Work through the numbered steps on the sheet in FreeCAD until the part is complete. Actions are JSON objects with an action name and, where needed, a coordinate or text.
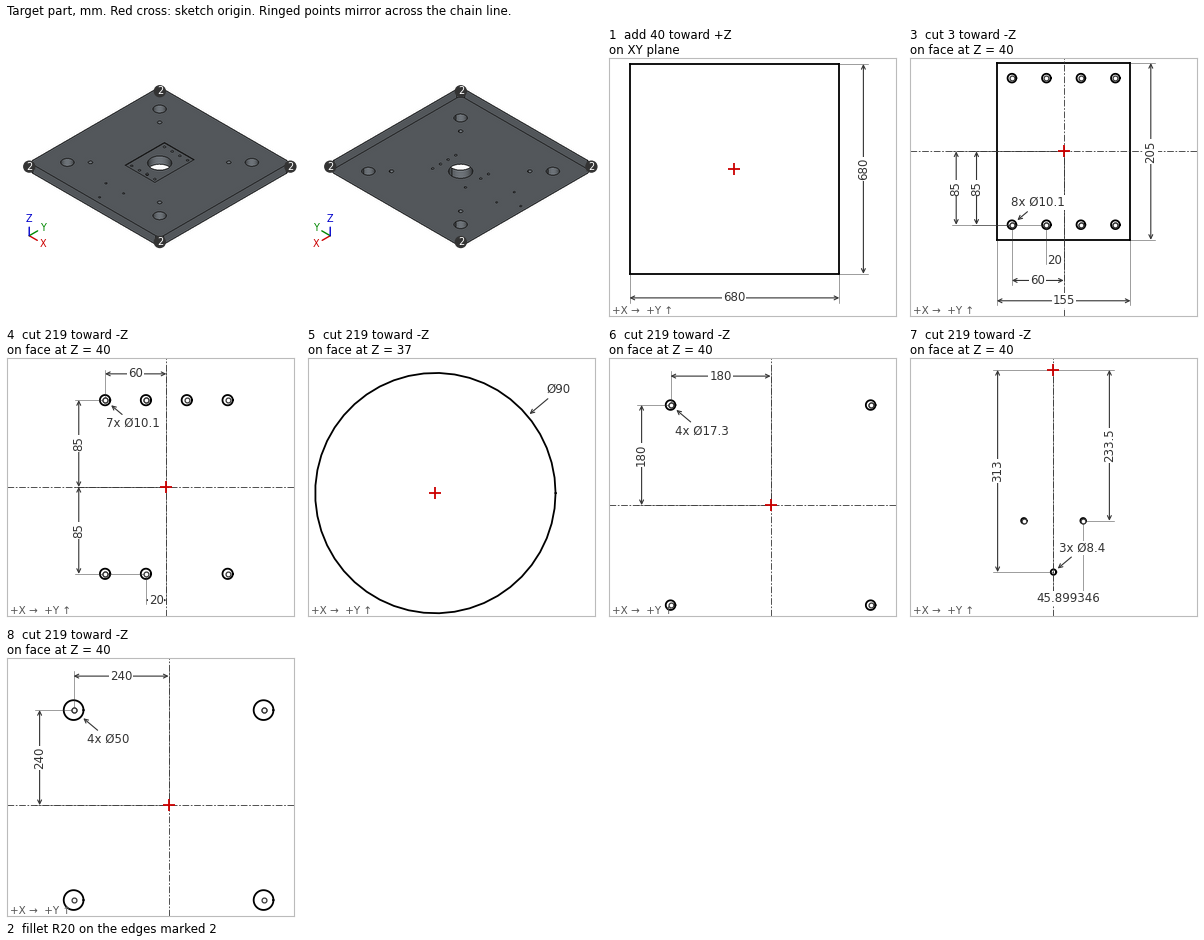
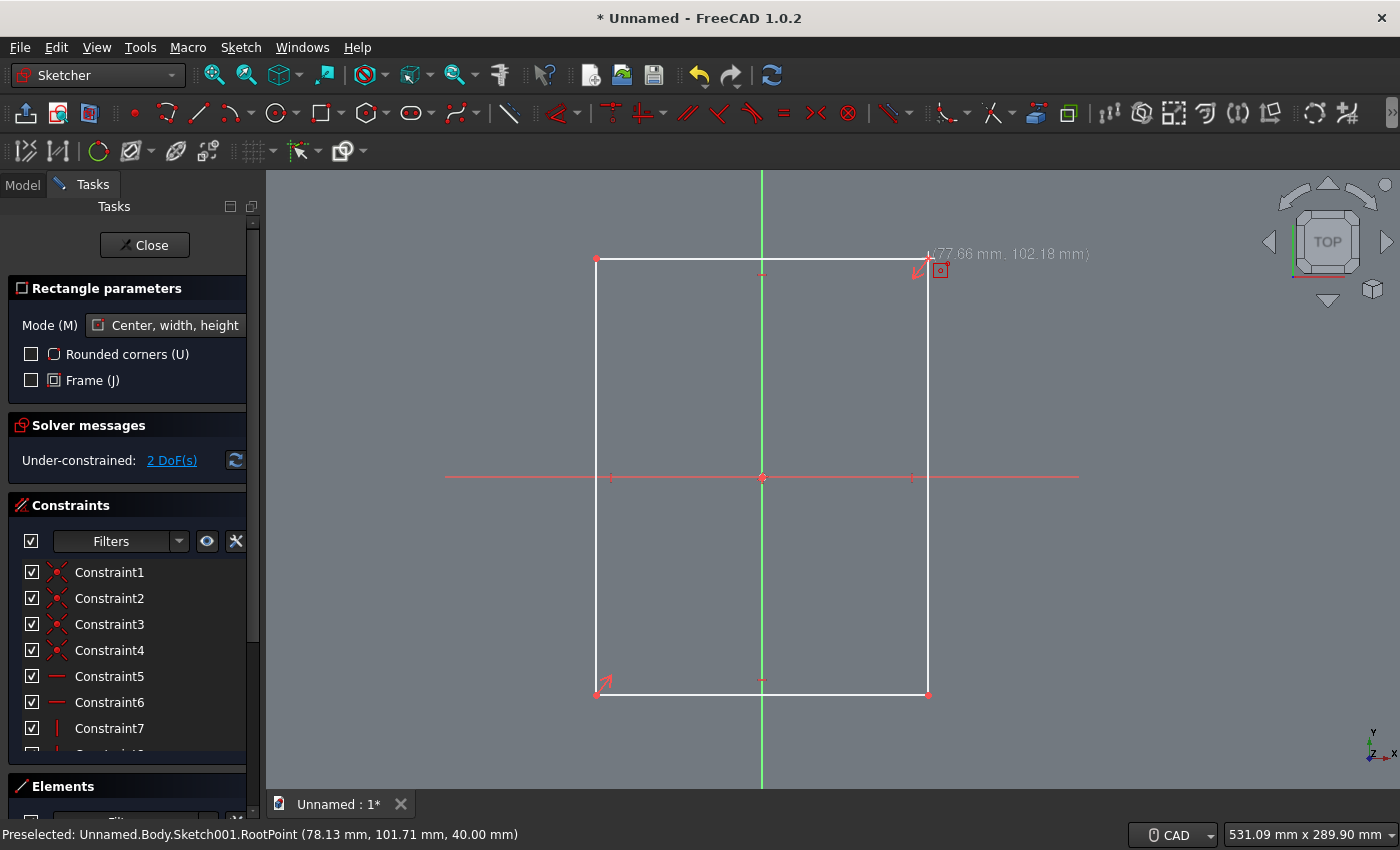
{"action": "left_click", "coordinate": [276, 114]}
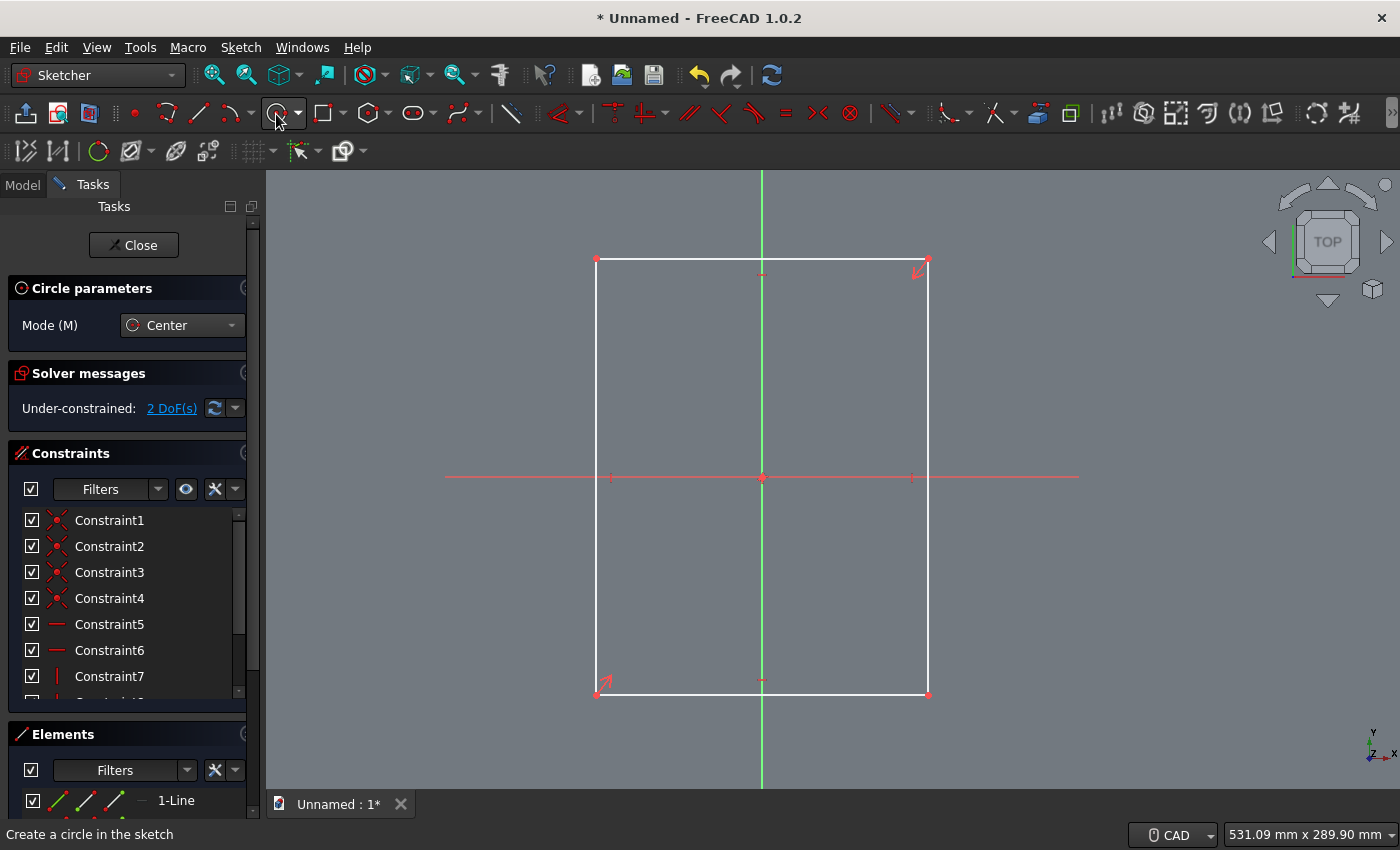
{"action": "scroll", "coordinate": [634, 659], "scroll_direction": "up", "scroll_amount": 4}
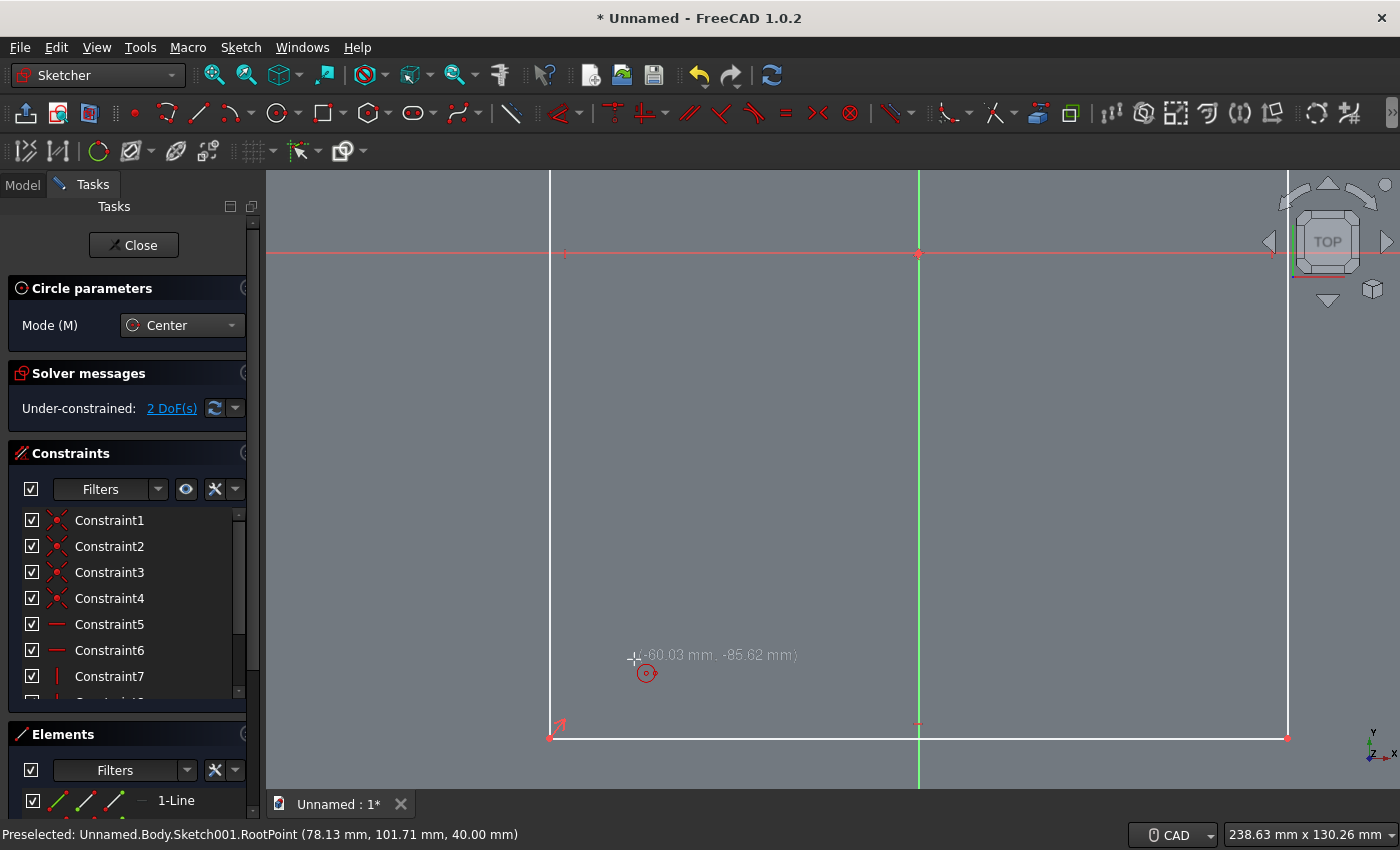
{"action": "left_click", "coordinate": [634, 657]}
{"action": "left_click", "coordinate": [651, 640]}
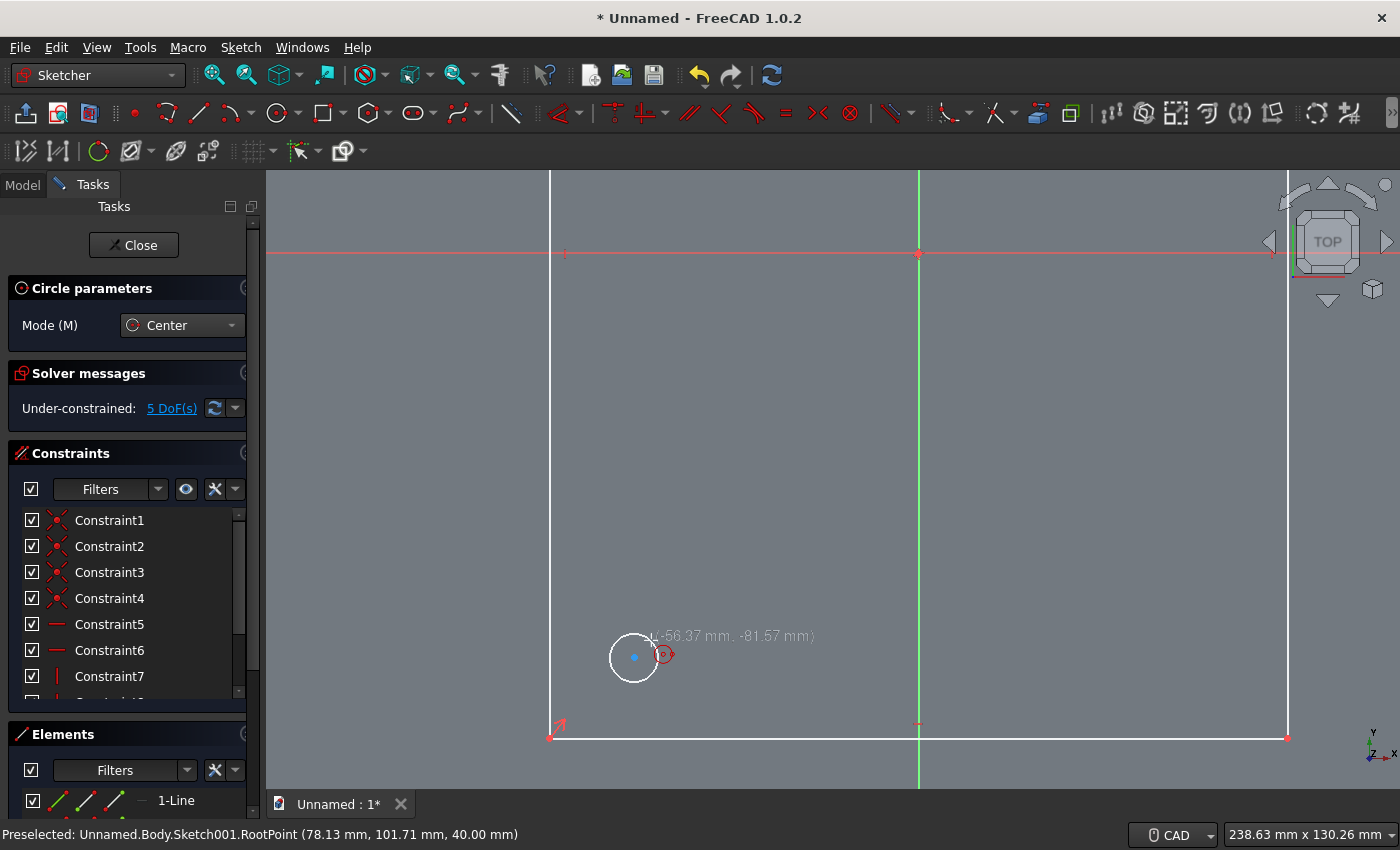
{"action": "left_click", "coordinate": [824, 657]}
{"action": "left_click", "coordinate": [841, 640]}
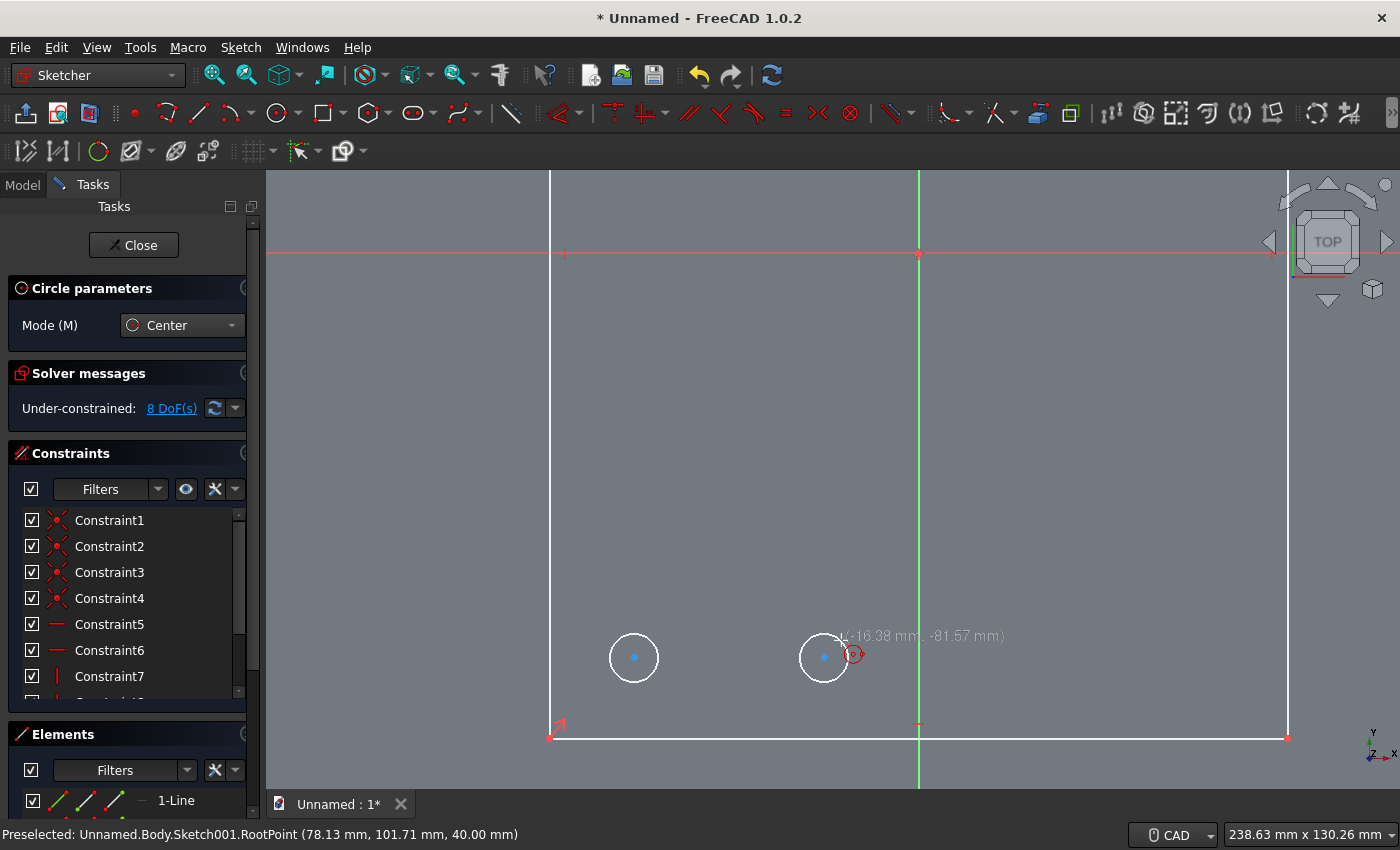
{"action": "left_click", "coordinate": [1014, 657]}
{"action": "left_click", "coordinate": [1031, 640]}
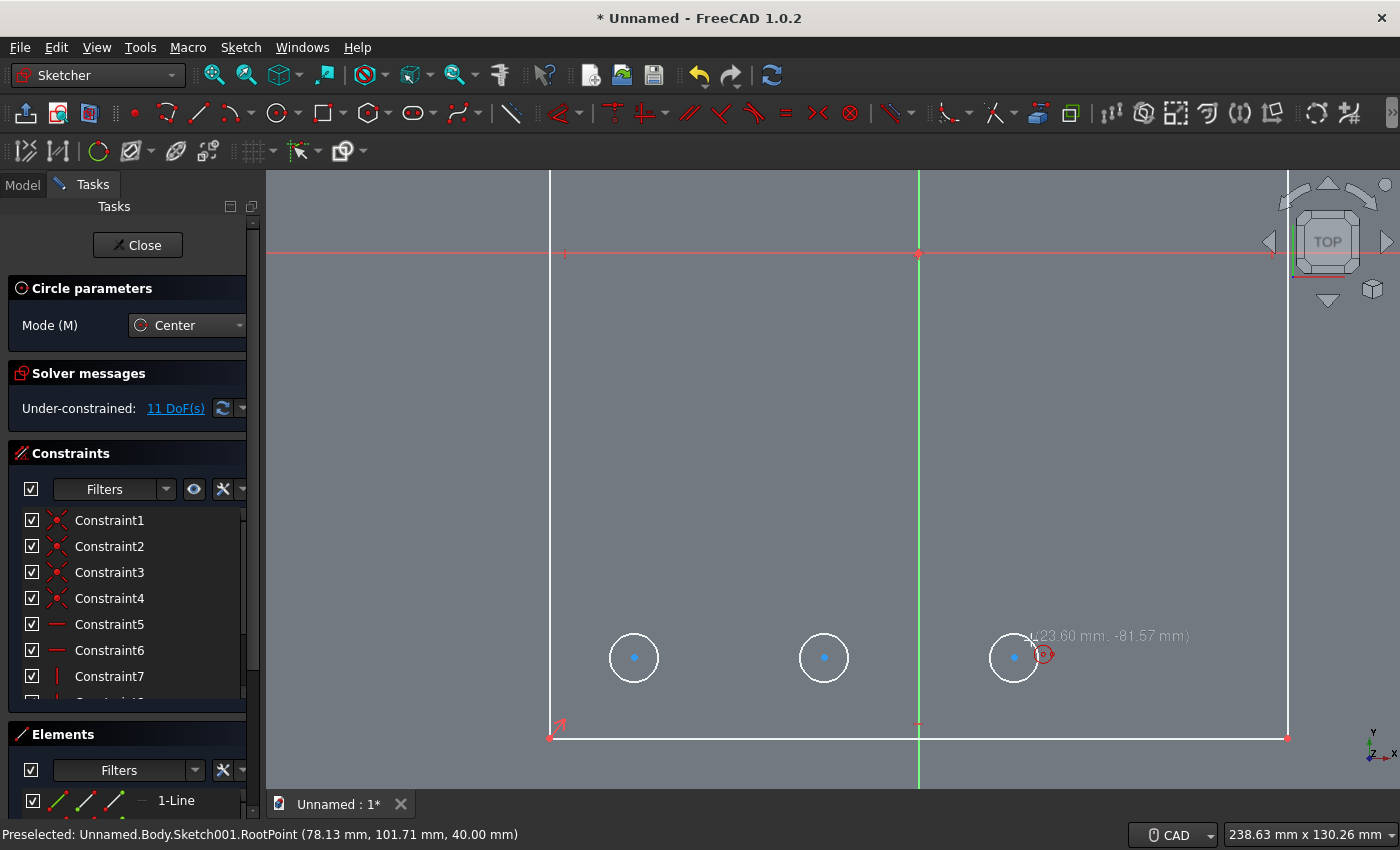
{"action": "left_click", "coordinate": [1204, 657]}
{"action": "left_click", "coordinate": [1221, 640]}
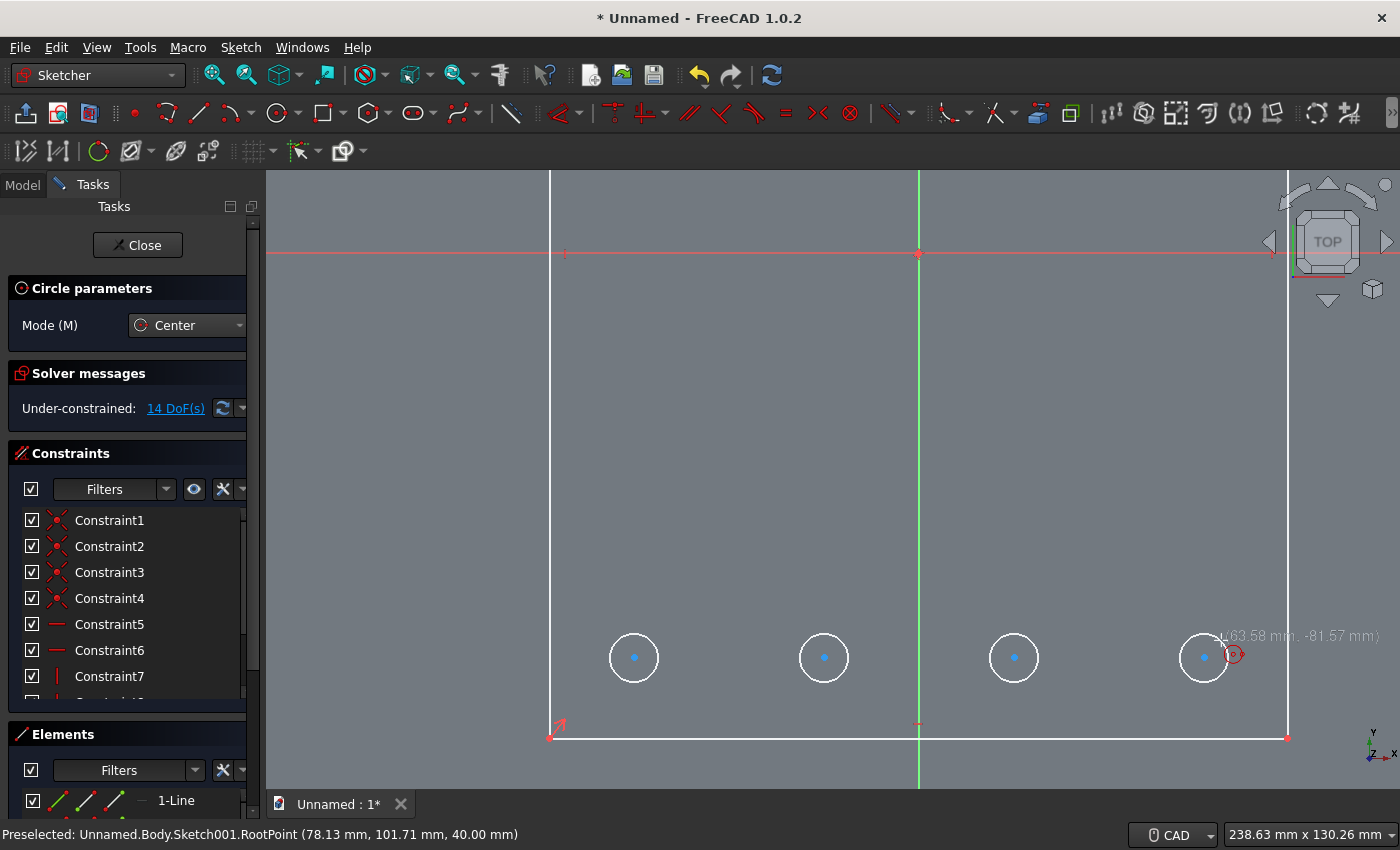
{"action": "scroll", "coordinate": [639, 664], "scroll_direction": "down", "scroll_amount": 4}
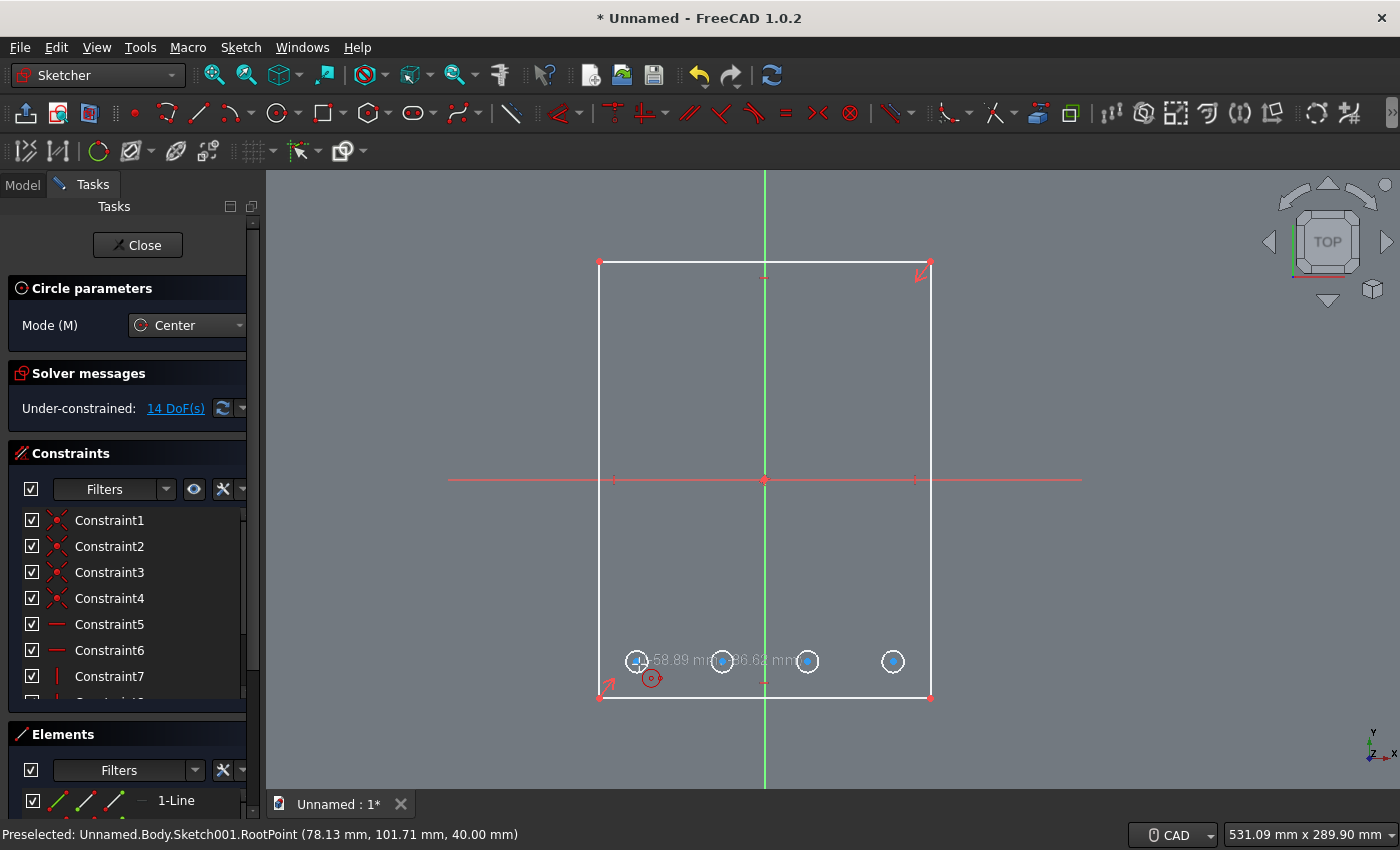
{"action": "scroll", "coordinate": [637, 298], "scroll_direction": "up", "scroll_amount": 4}